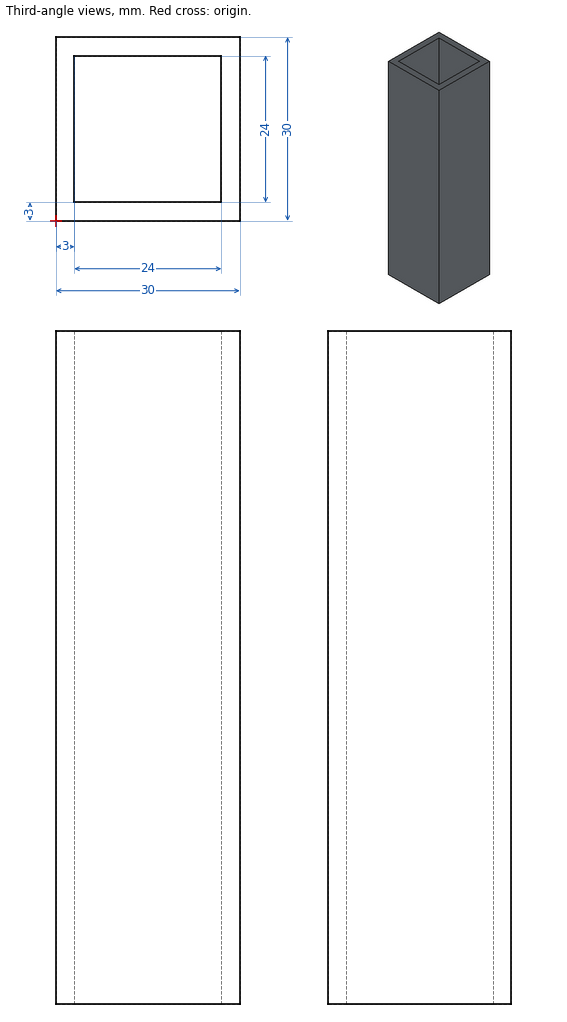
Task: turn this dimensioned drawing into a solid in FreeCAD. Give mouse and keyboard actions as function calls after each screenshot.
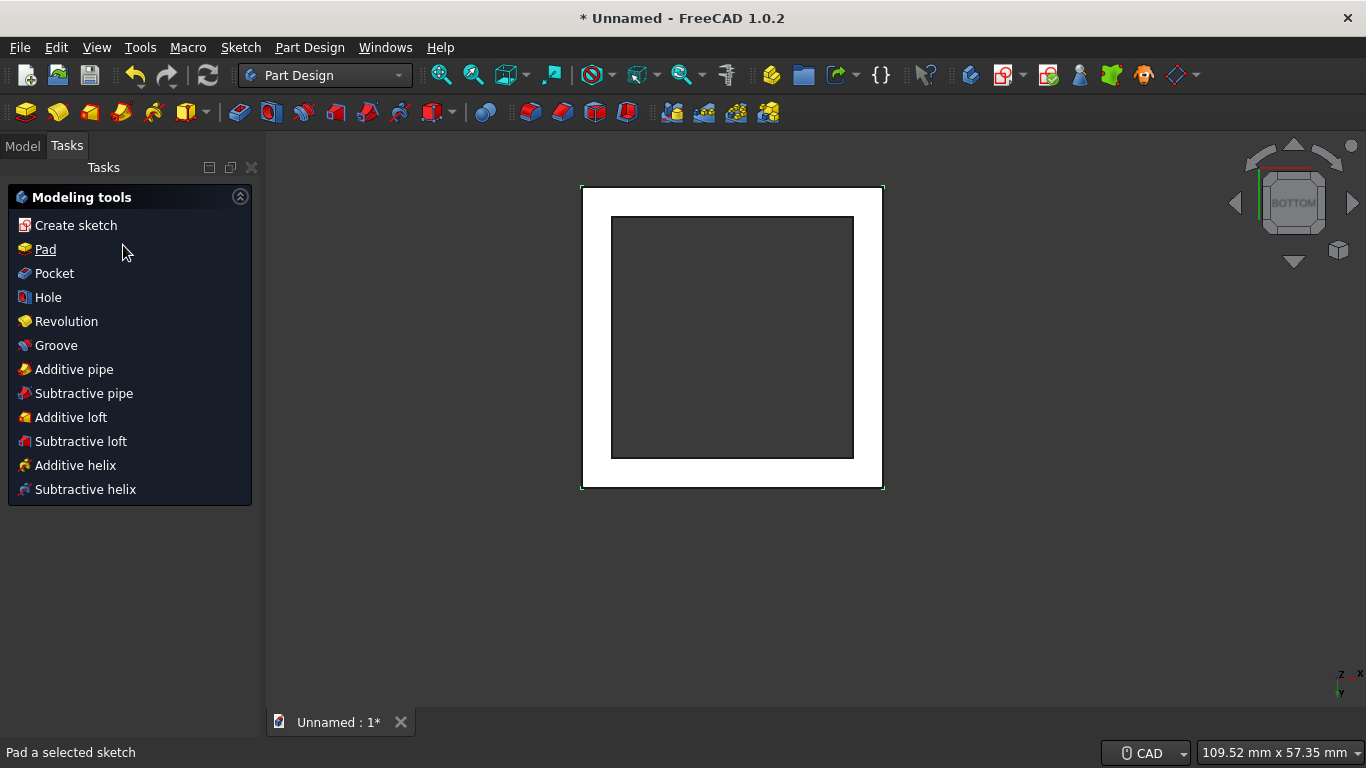
click(240, 112)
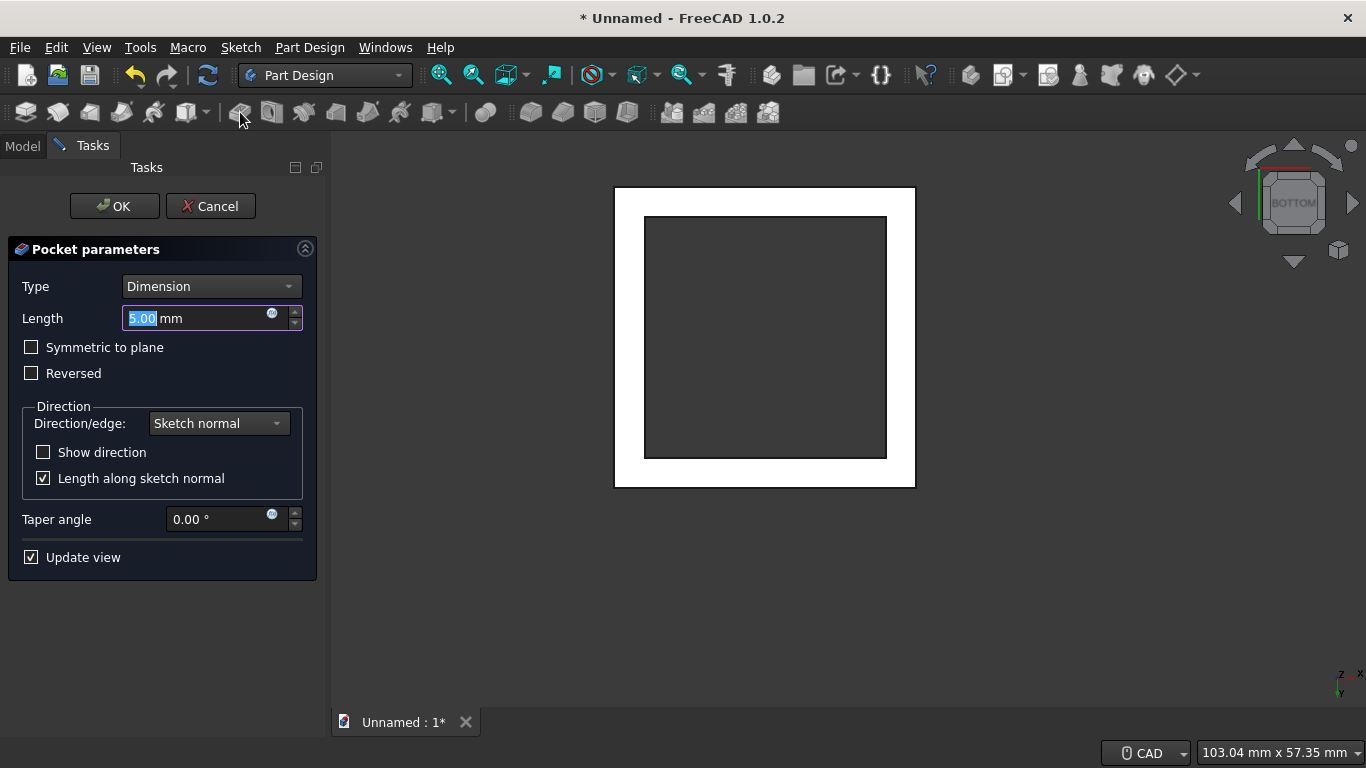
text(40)
key(Tab)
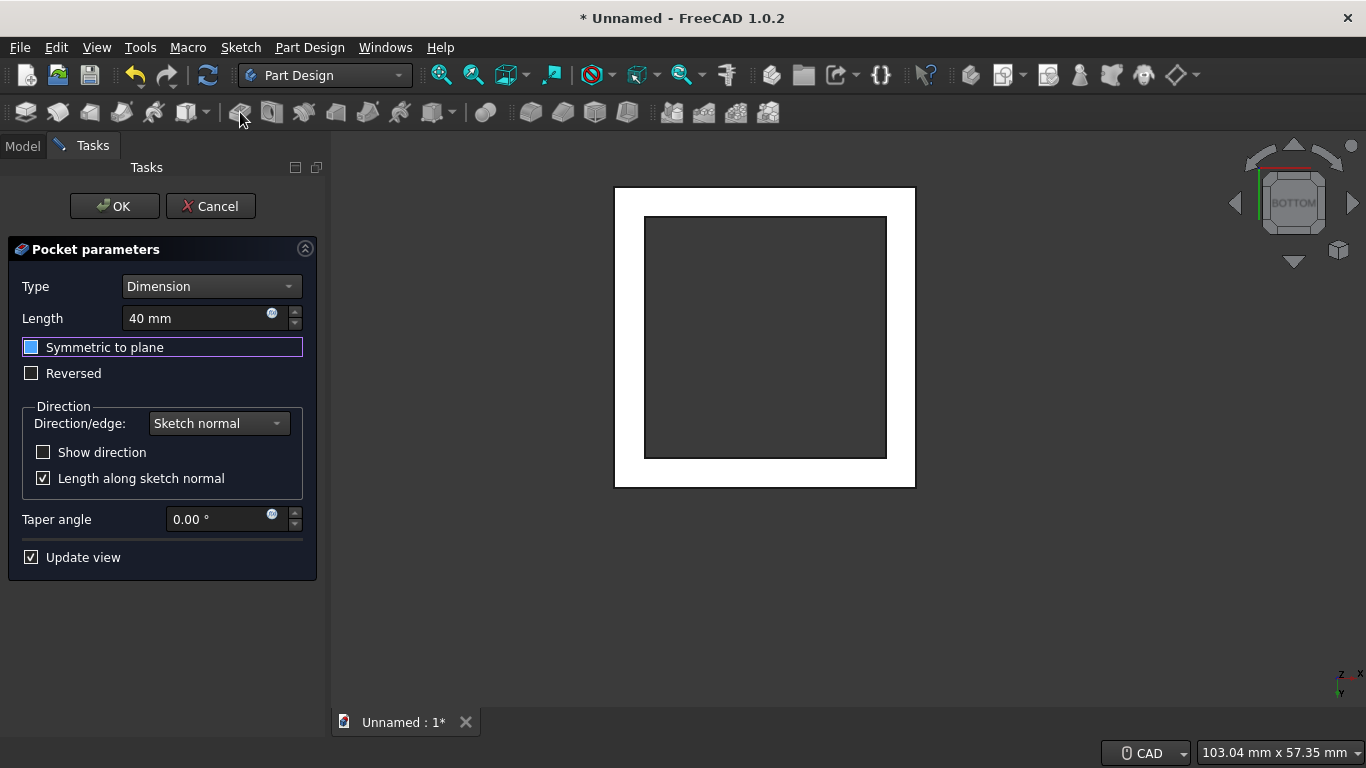
click(115, 206)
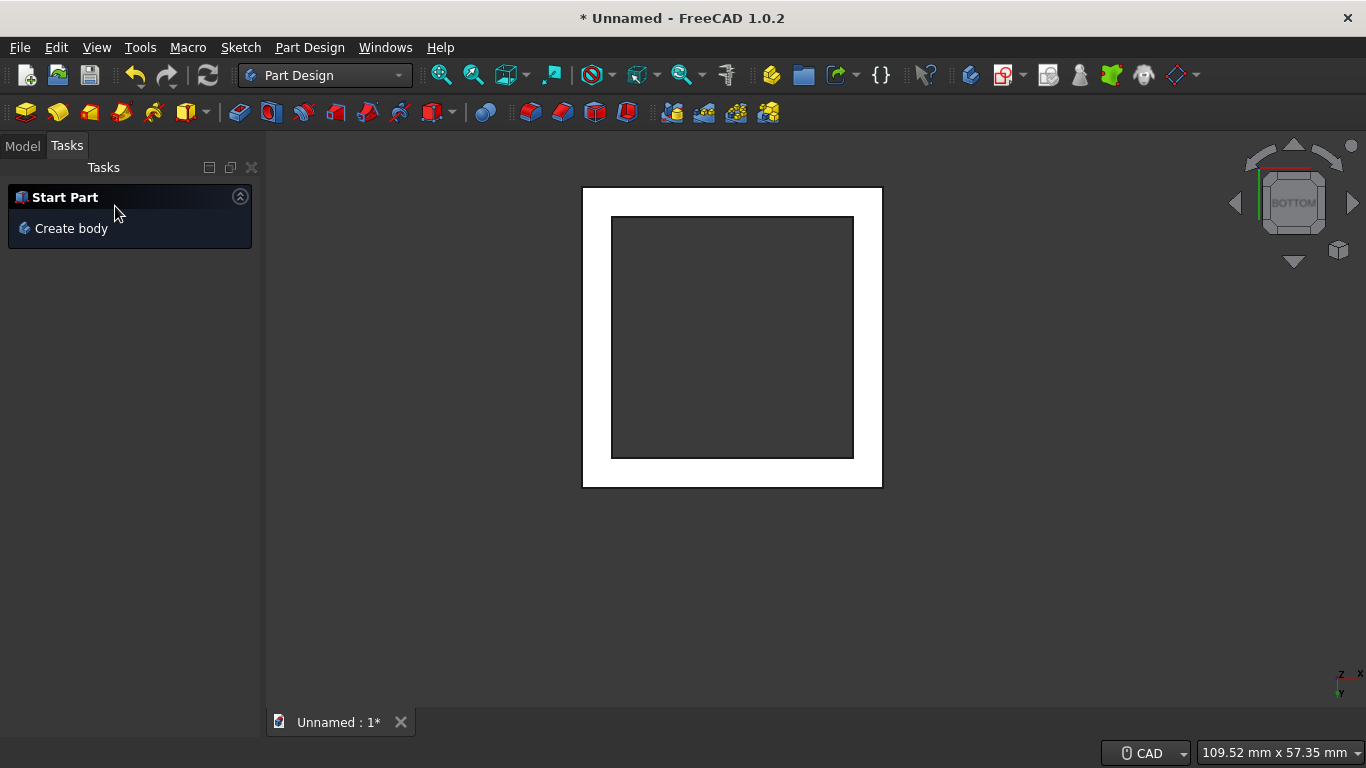
key(0)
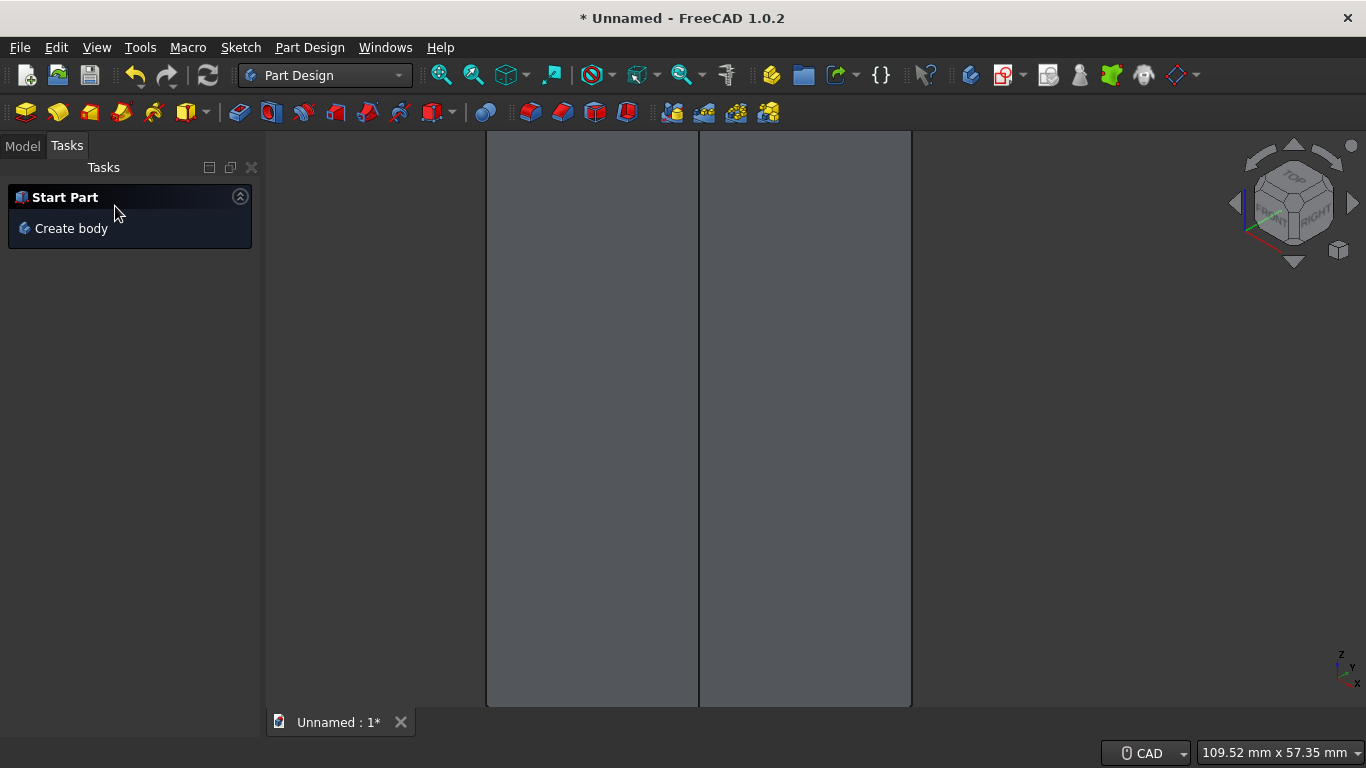
click(442, 76)